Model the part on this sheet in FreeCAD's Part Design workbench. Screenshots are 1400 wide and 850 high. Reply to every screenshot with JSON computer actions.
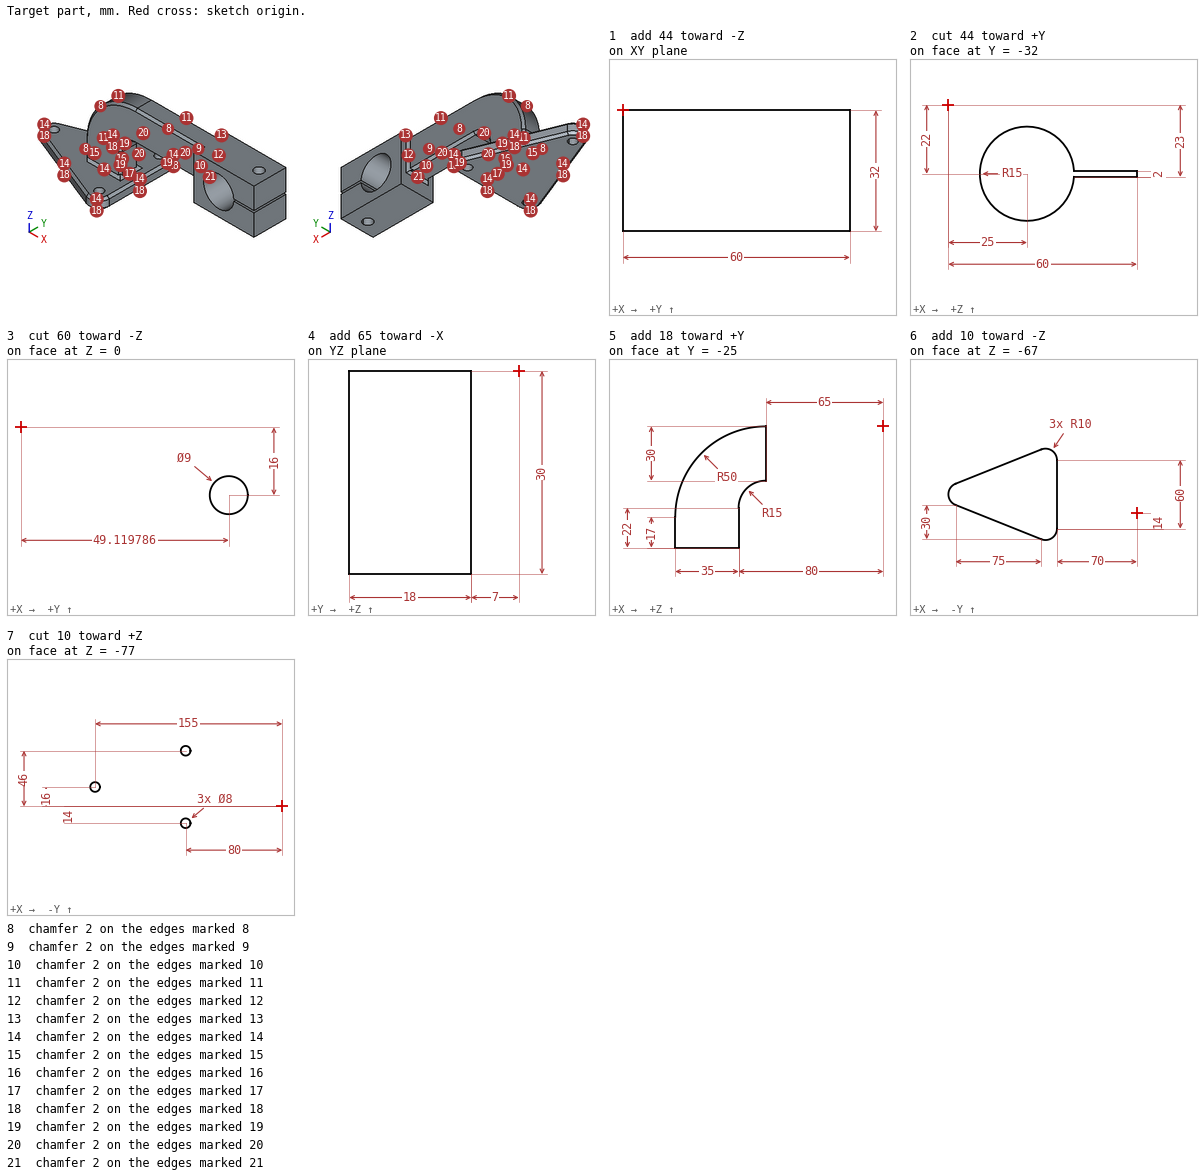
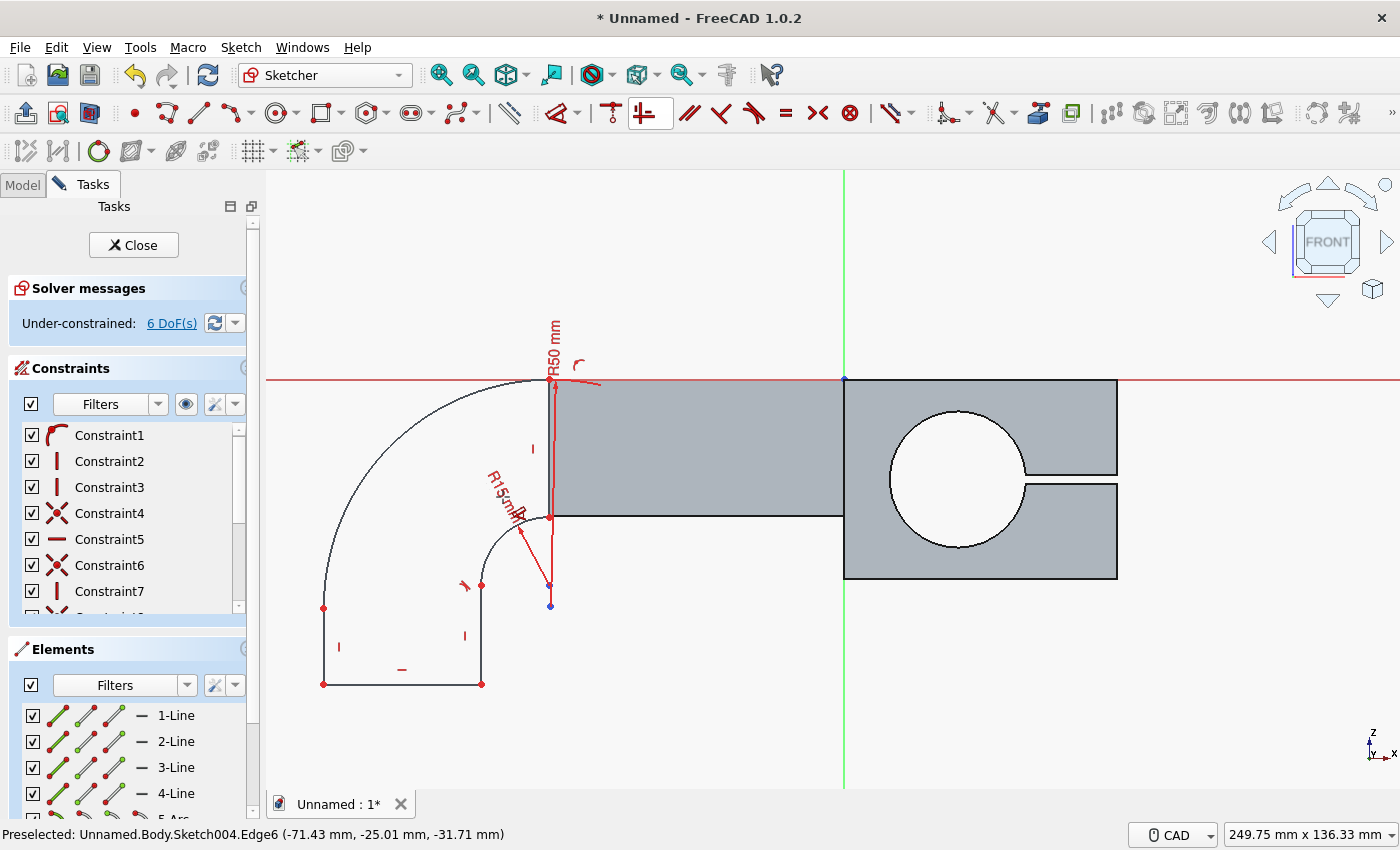
{"action": "left_click", "coordinate": [549, 476]}
{"action": "left_click", "coordinate": [515, 448]}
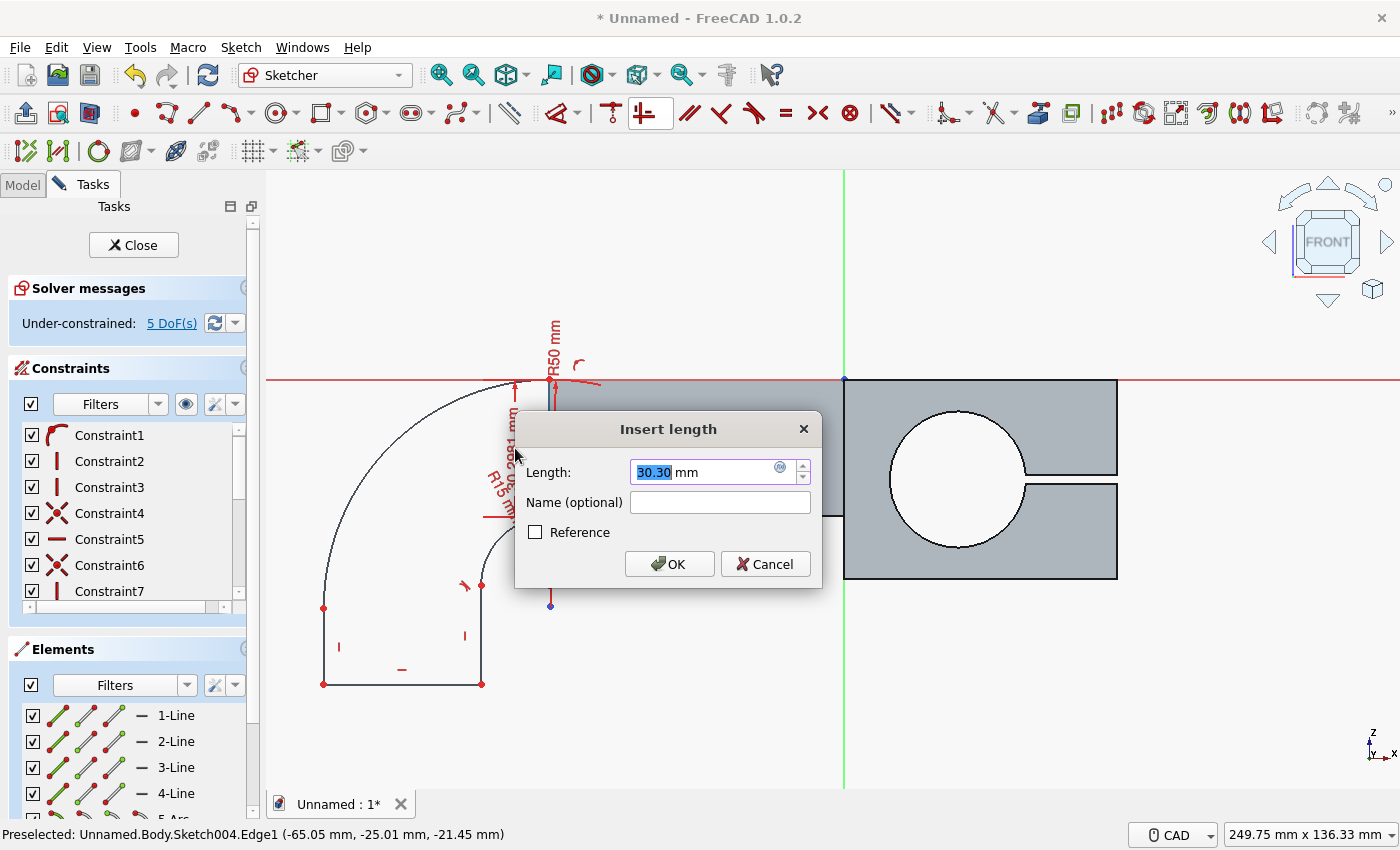
{"action": "type", "text": "30"}
{"action": "key", "text": "Return"}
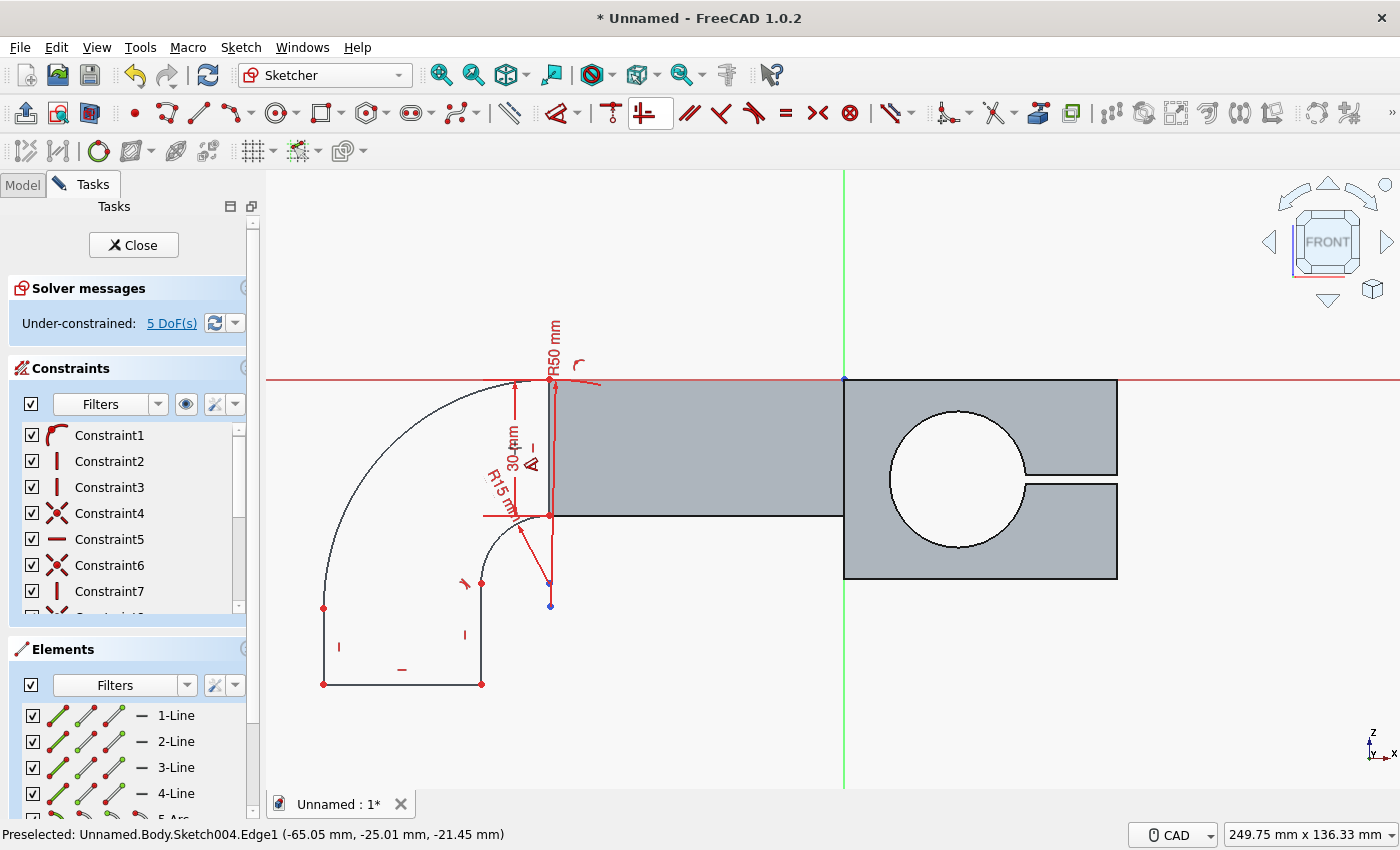
{"action": "left_click", "coordinate": [324, 631]}
{"action": "left_click", "coordinate": [358, 647]}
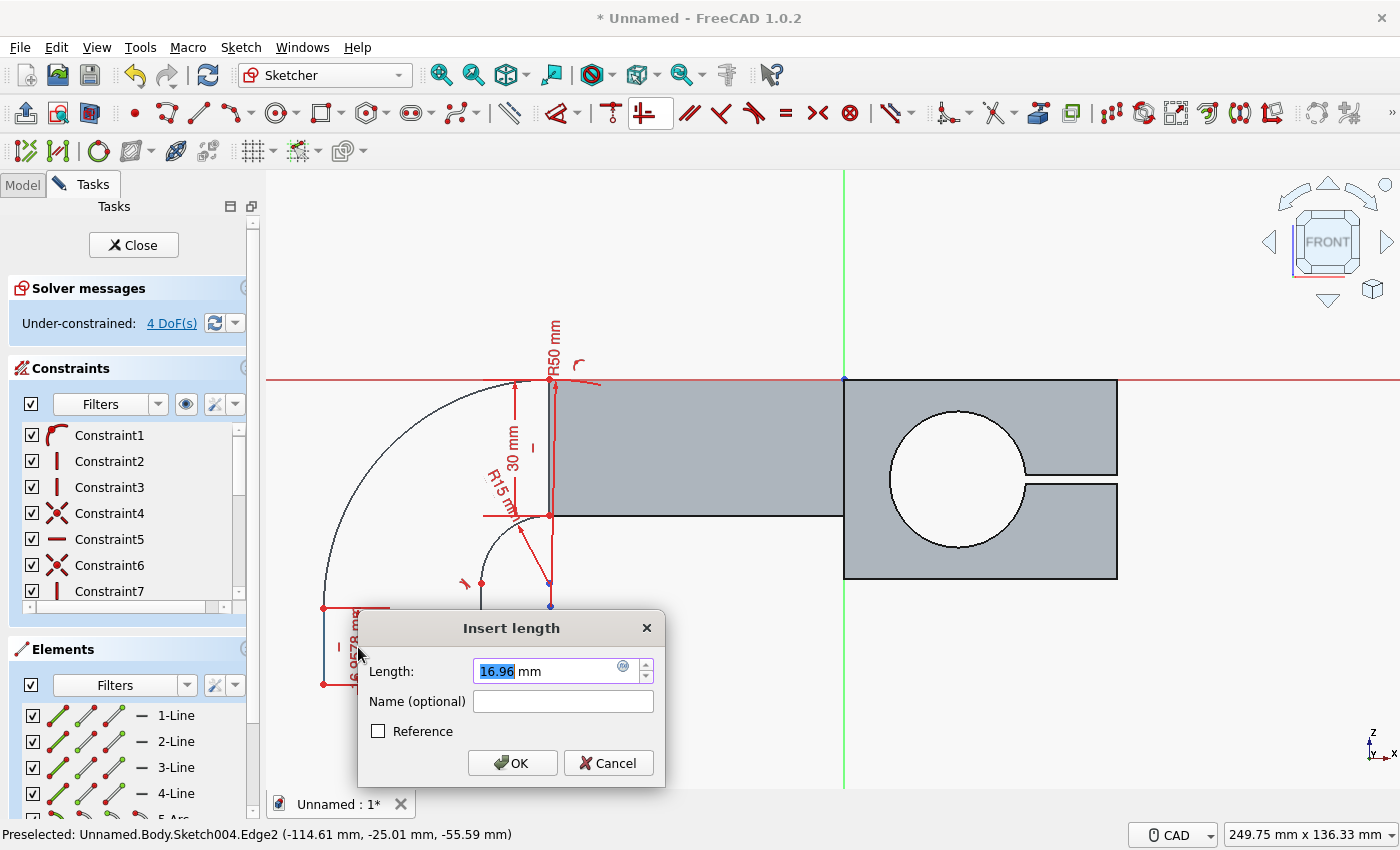
{"action": "type", "text": "17"}
{"action": "key", "text": "Return"}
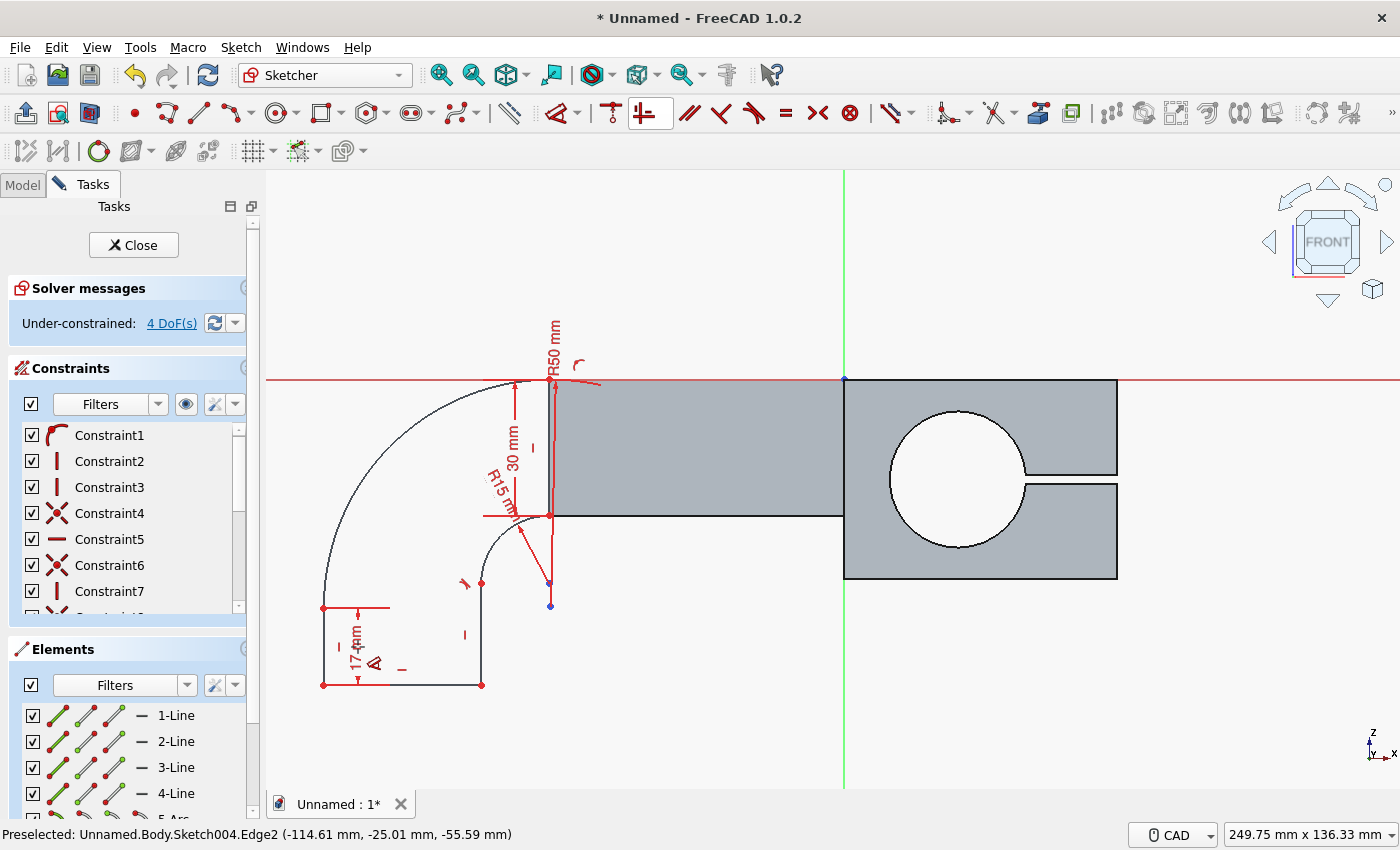
{"action": "left_click", "coordinate": [371, 685]}
{"action": "left_click", "coordinate": [403, 719]}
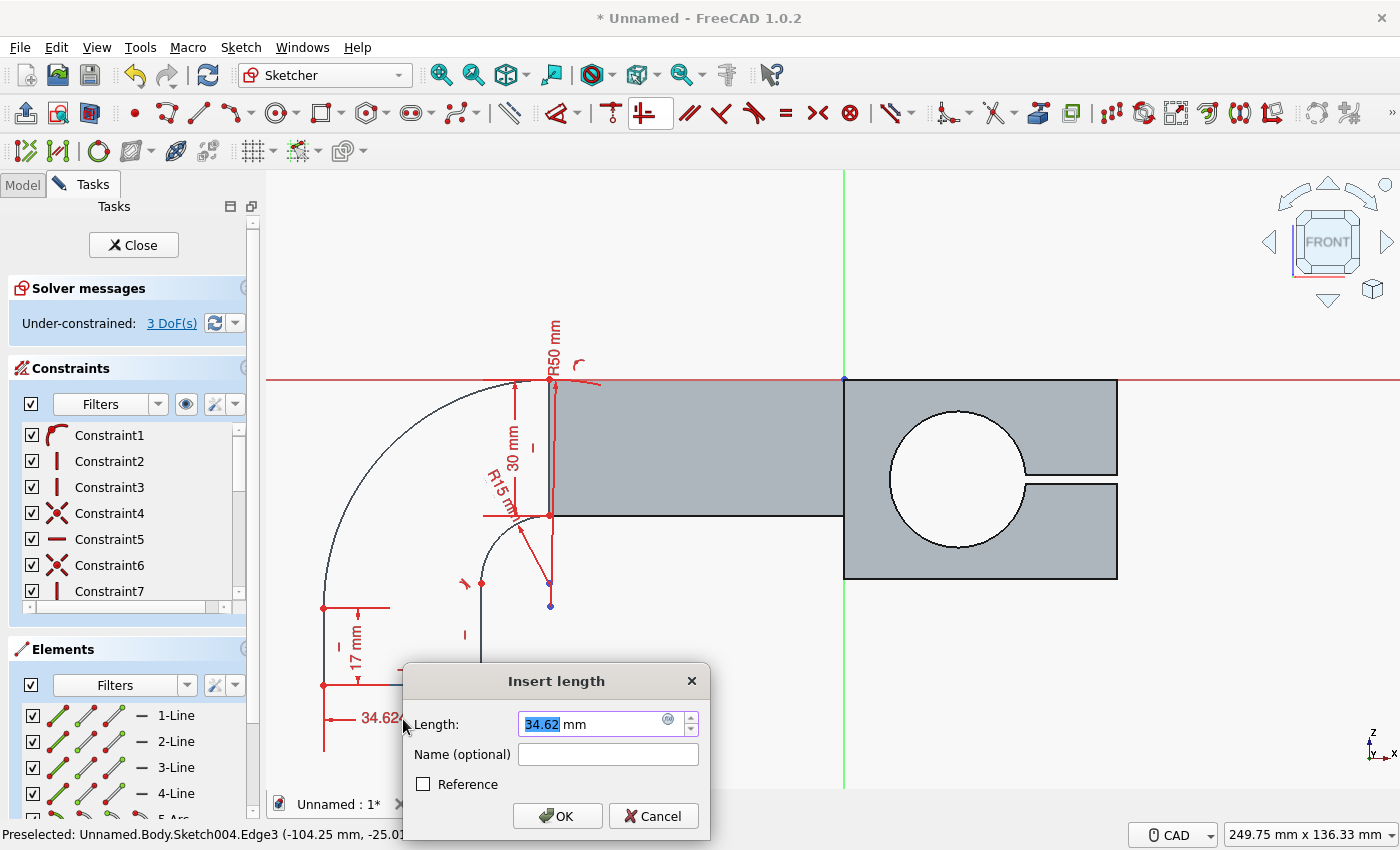
{"action": "type", "text": "35"}
{"action": "key", "text": "Return"}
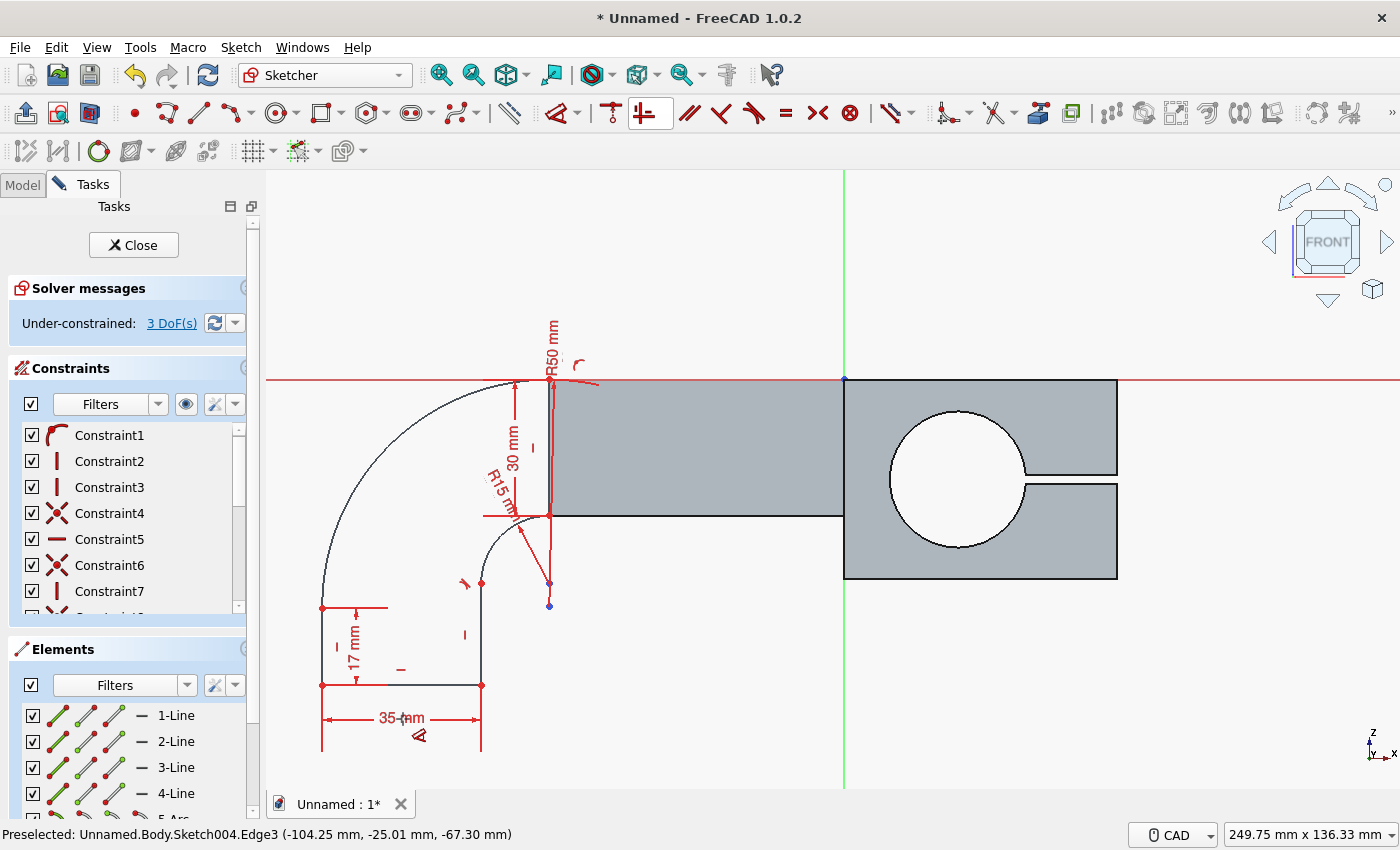
{"action": "left_click", "coordinate": [481, 655]}
{"action": "left_click", "coordinate": [447, 635]}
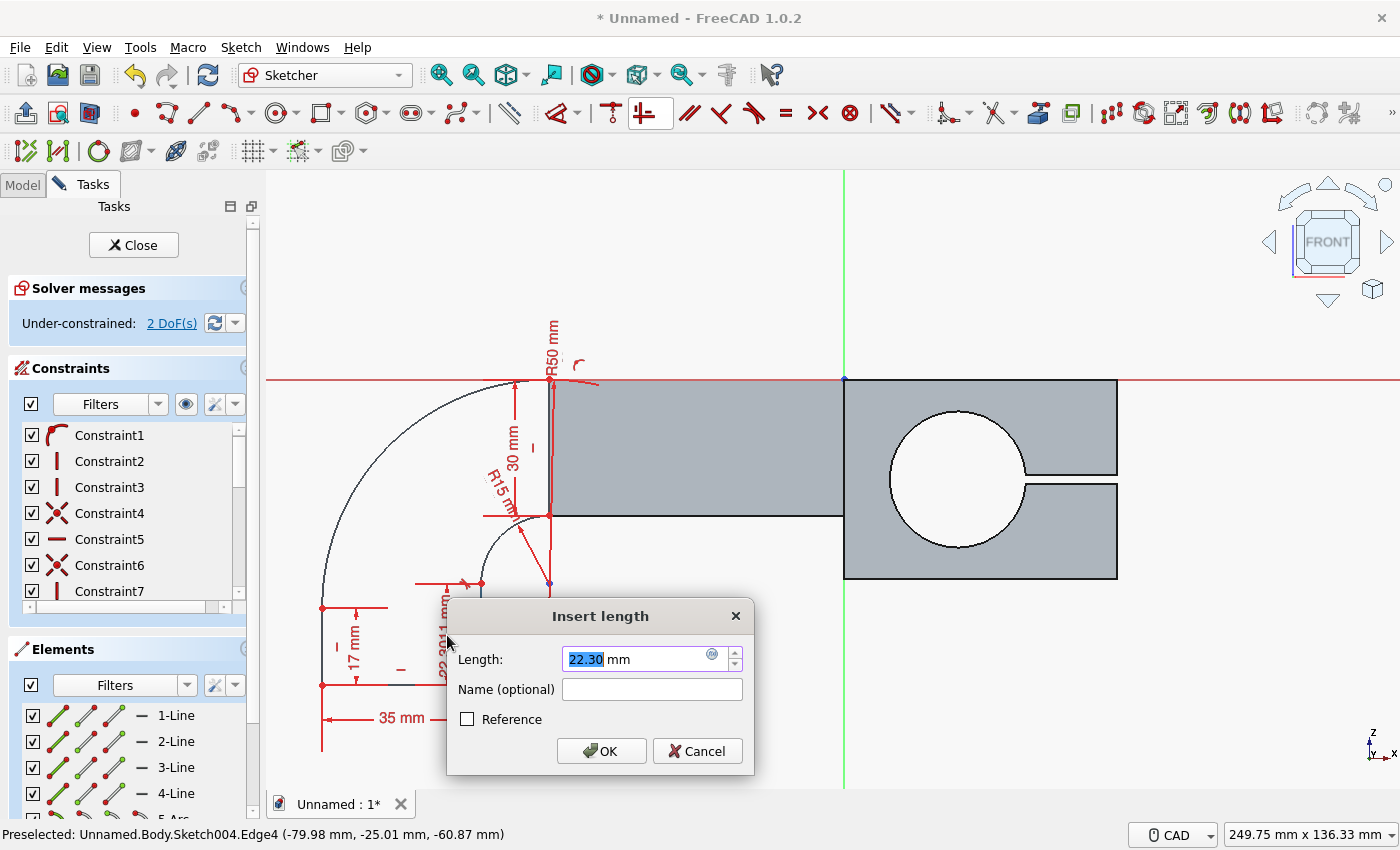
{"action": "type", "text": "22"}
{"action": "key", "text": "Return"}